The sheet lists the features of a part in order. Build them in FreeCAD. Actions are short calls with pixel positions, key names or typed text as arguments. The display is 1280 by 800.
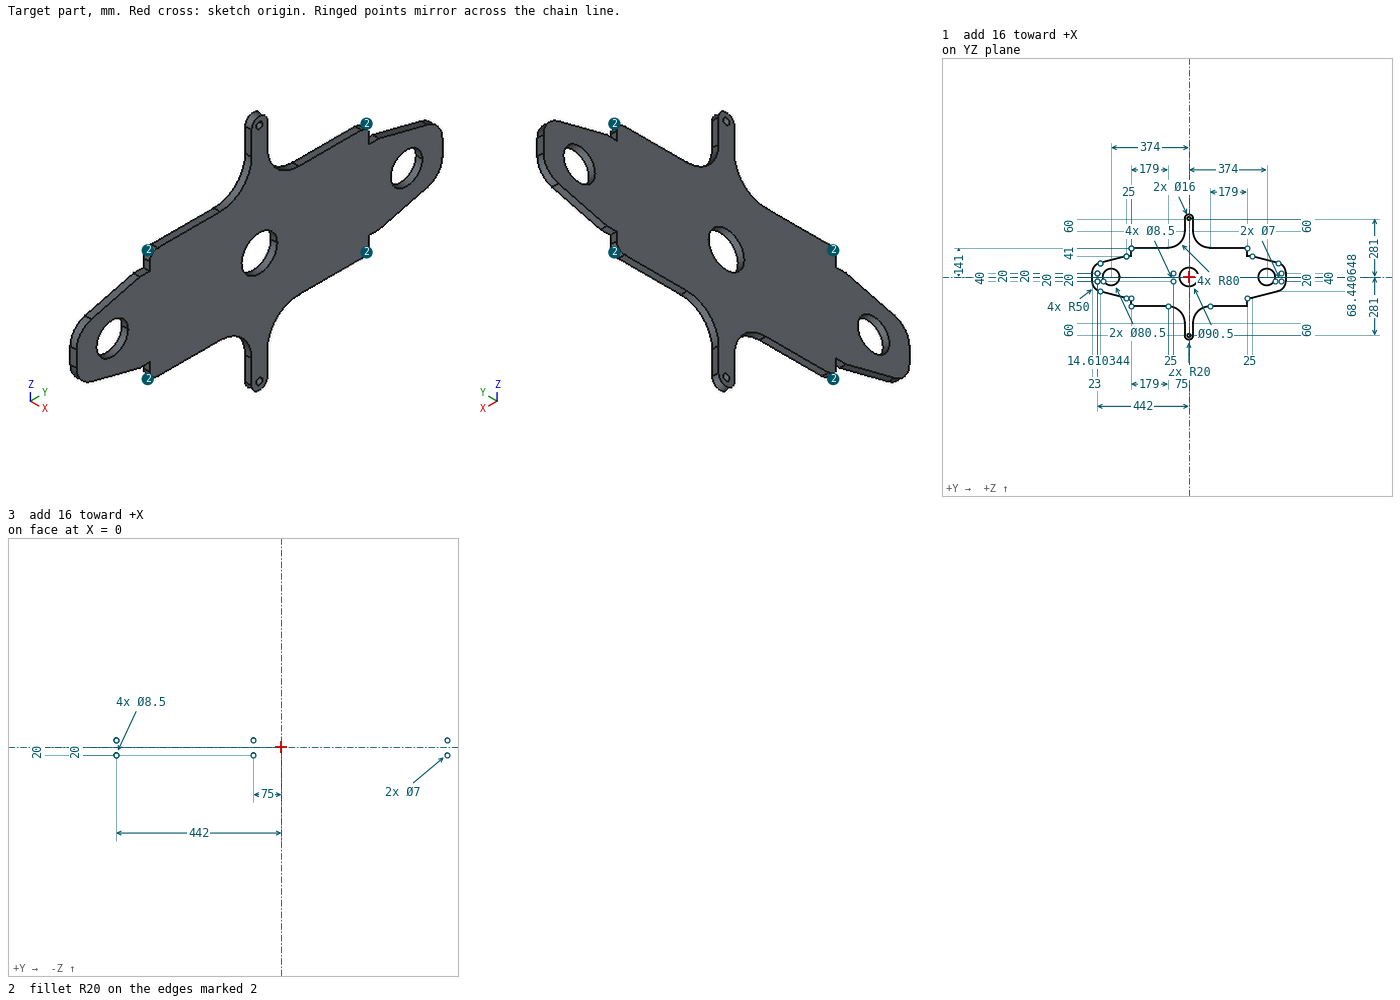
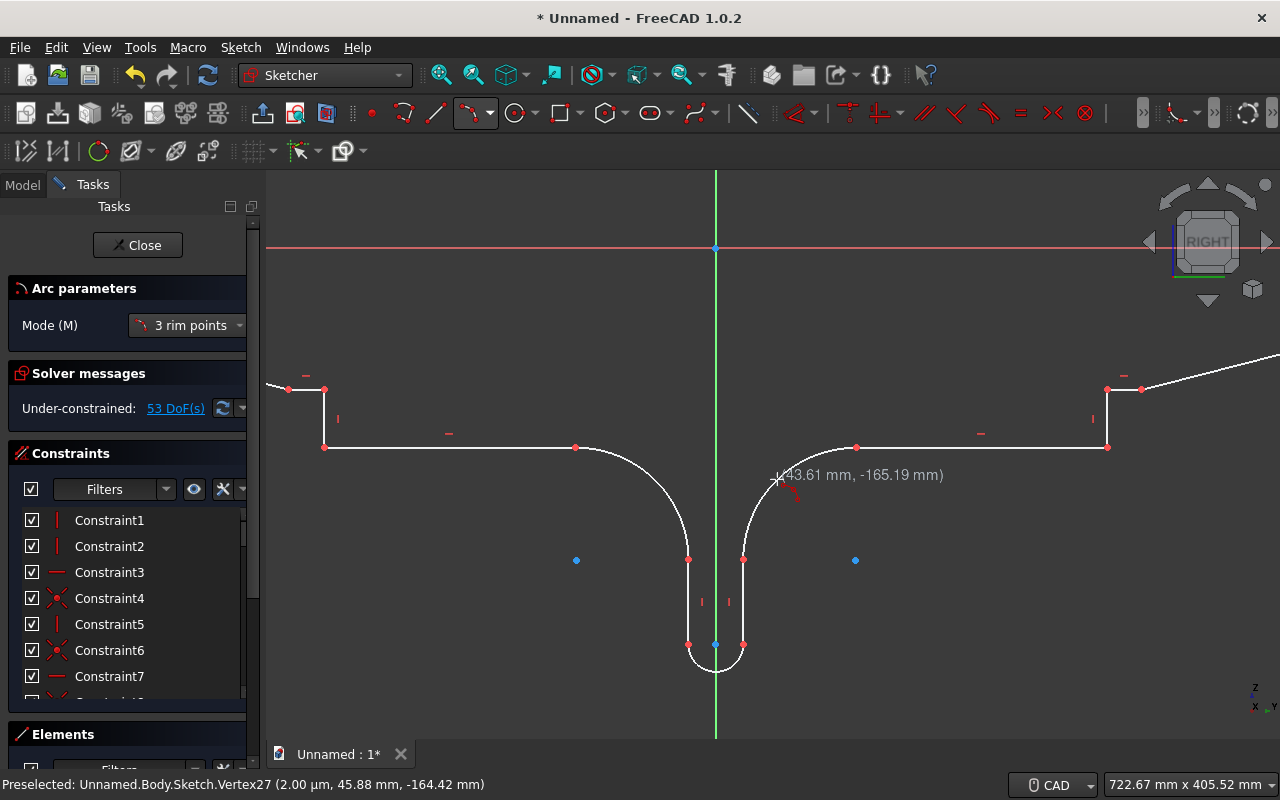
scroll(695, 623, down, 4)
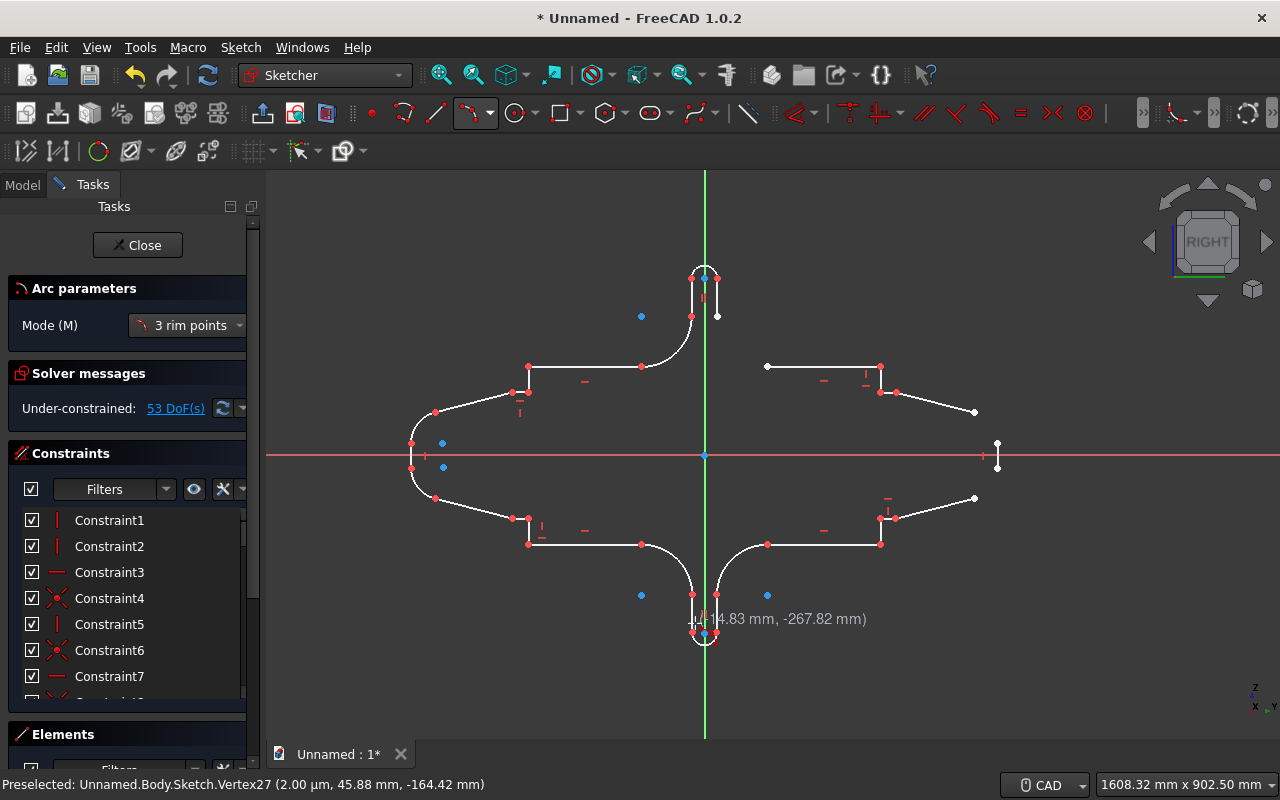
click(974, 499)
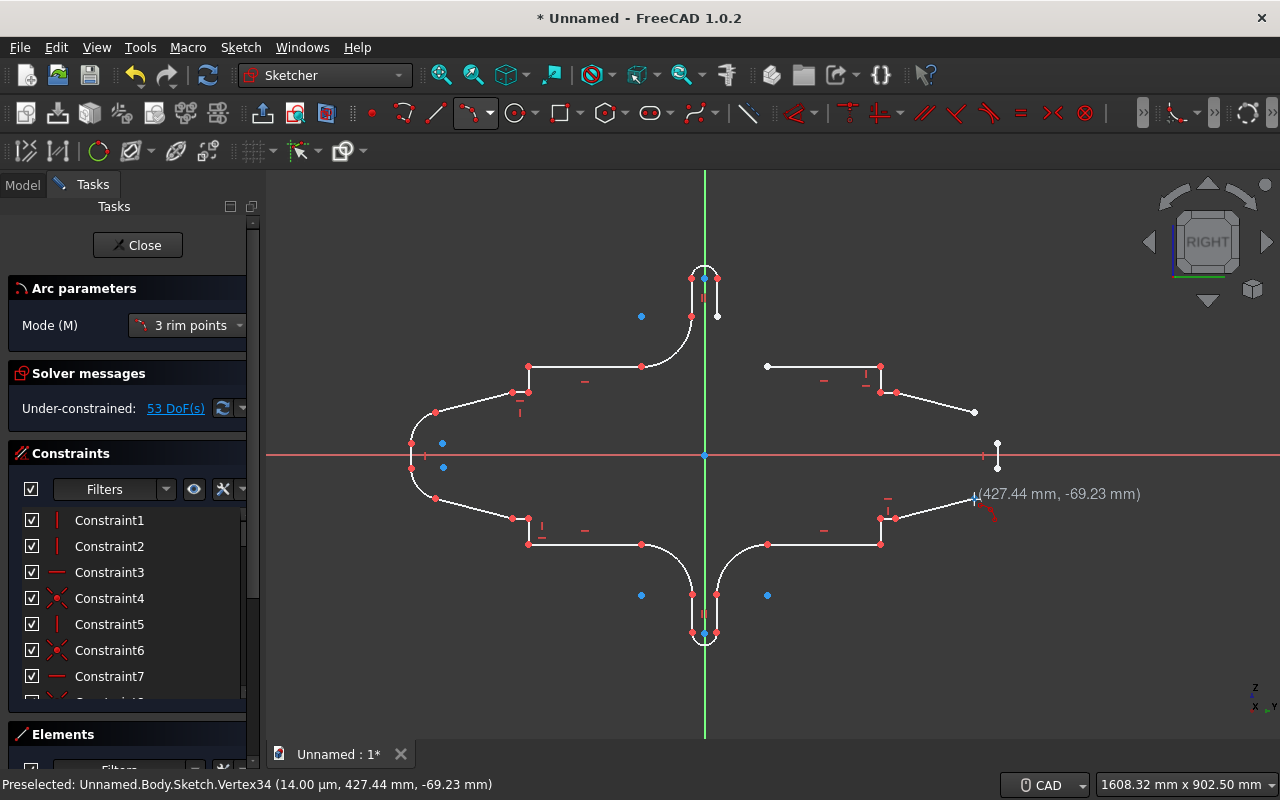
scroll(998, 468, up, 2)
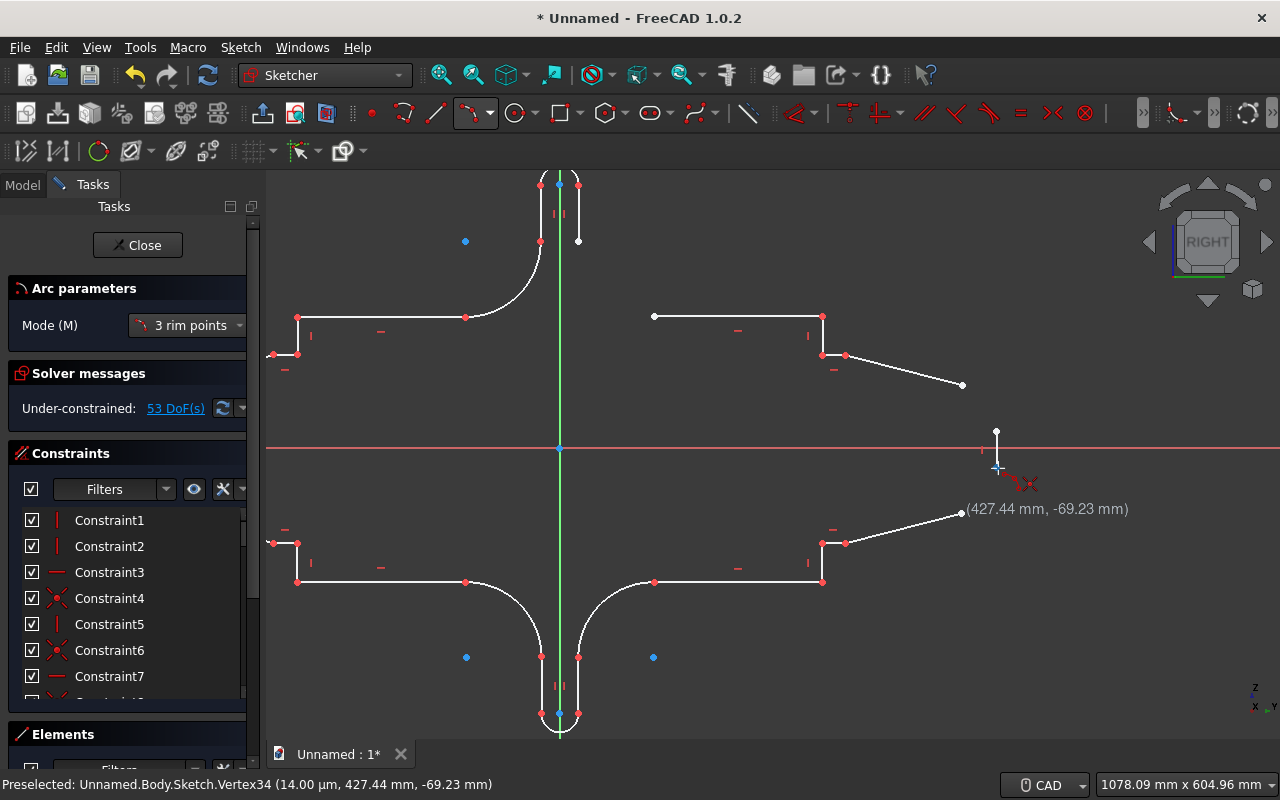
click(997, 468)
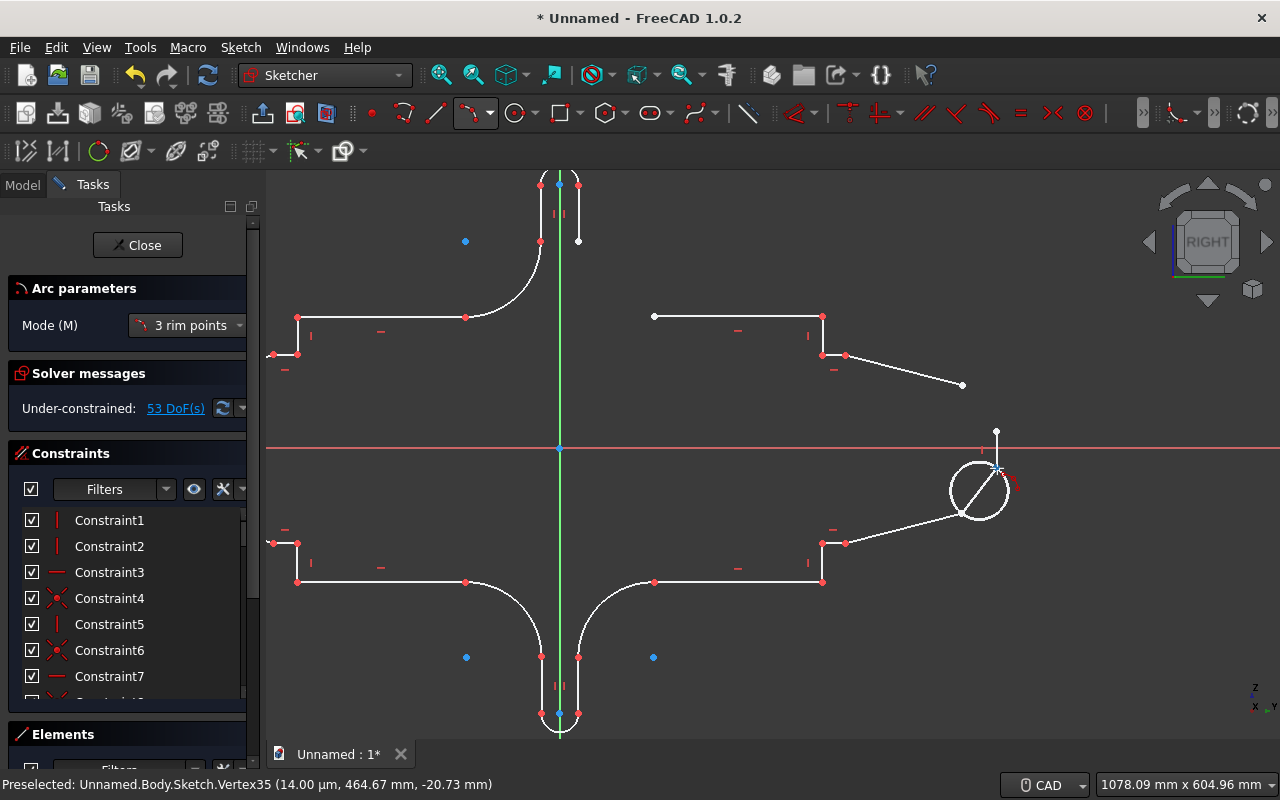
scroll(987, 496, up, 3)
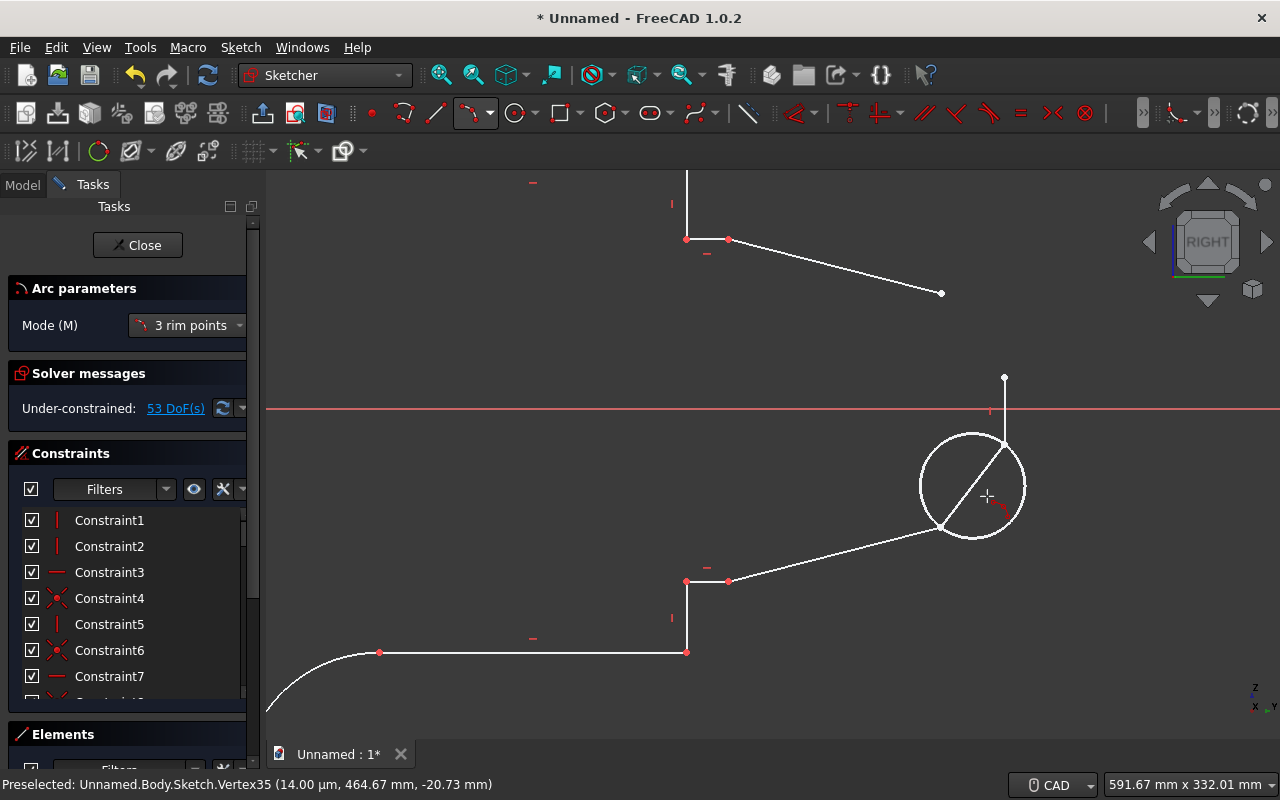
click(987, 496)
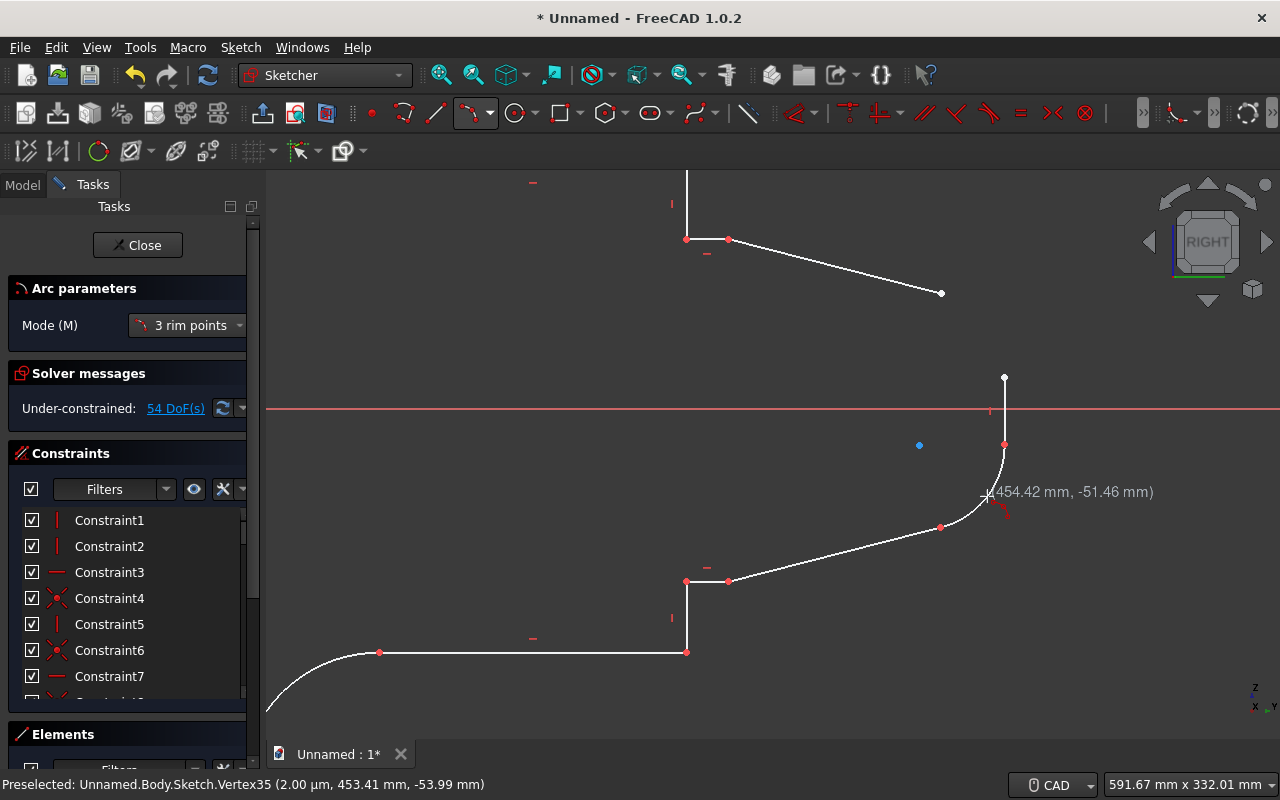
click(1005, 377)
click(941, 294)
click(987, 322)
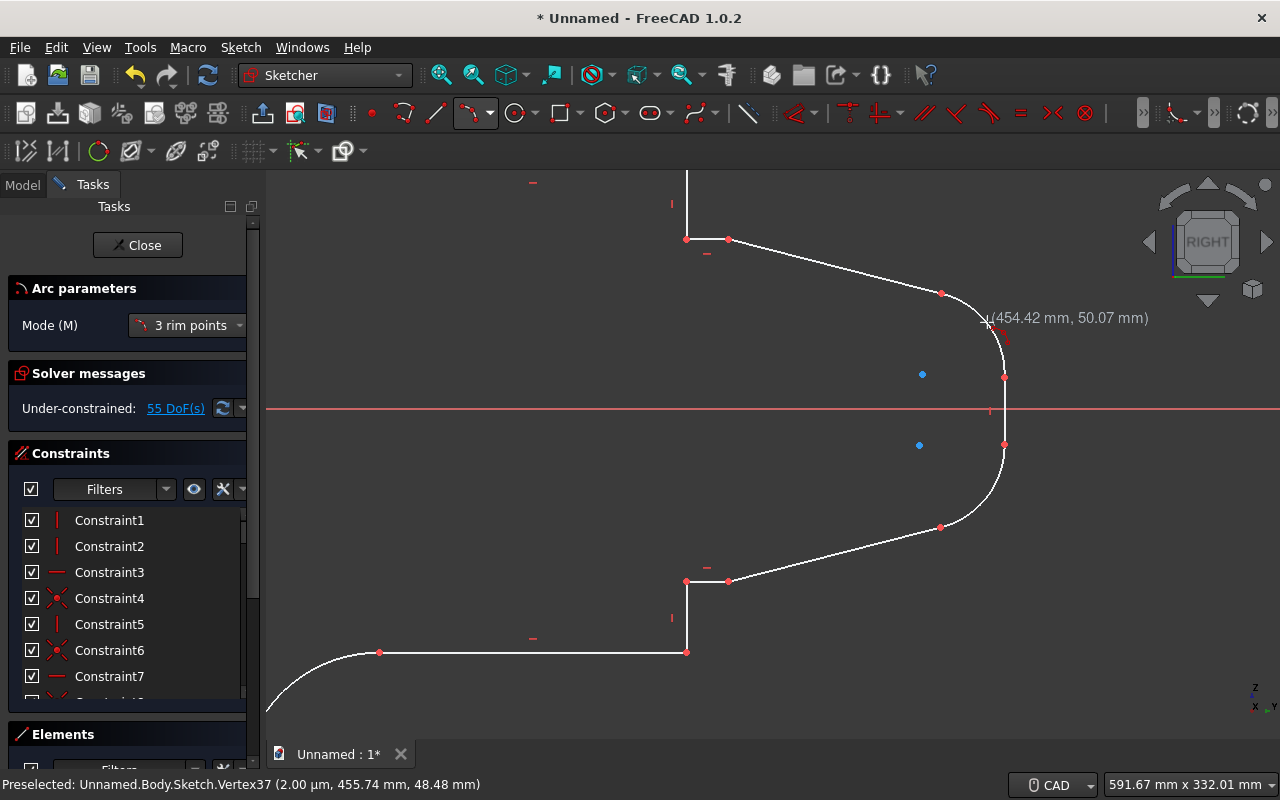
scroll(993, 481, down, 5)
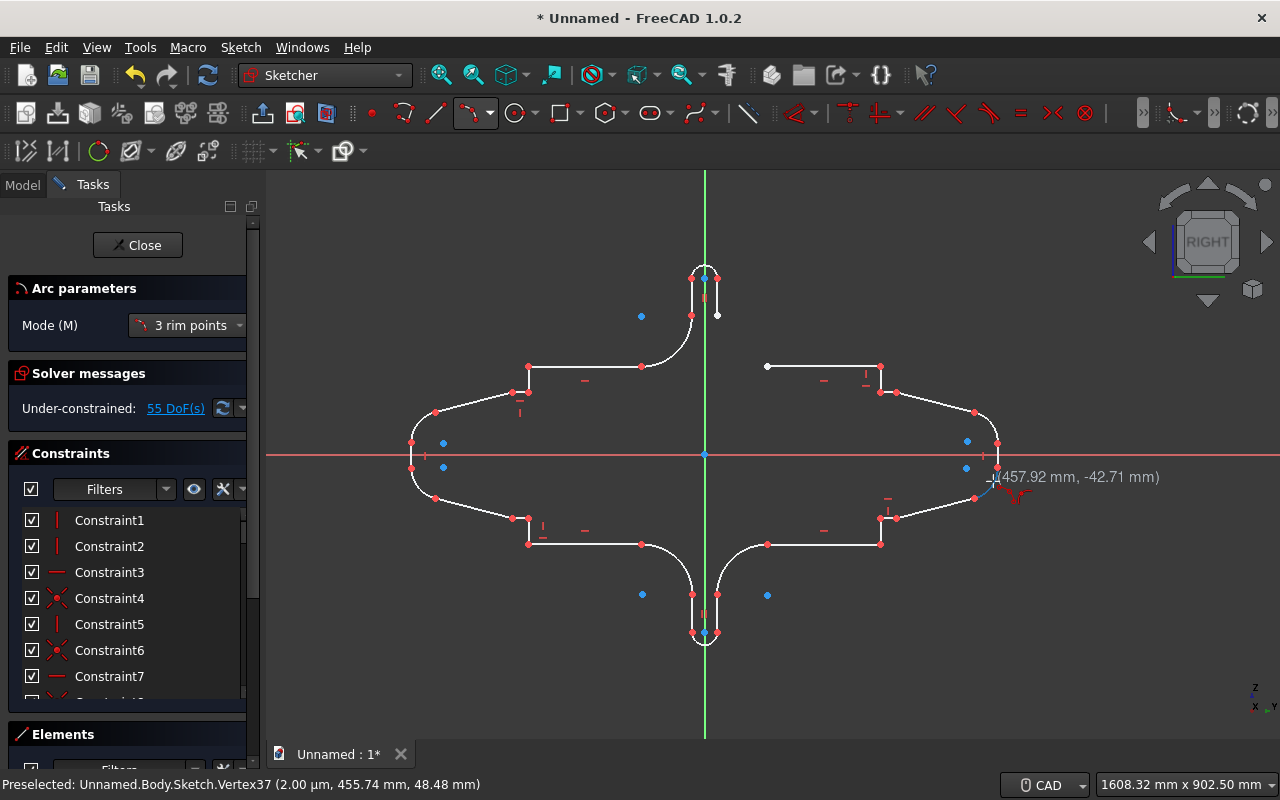
click(768, 366)